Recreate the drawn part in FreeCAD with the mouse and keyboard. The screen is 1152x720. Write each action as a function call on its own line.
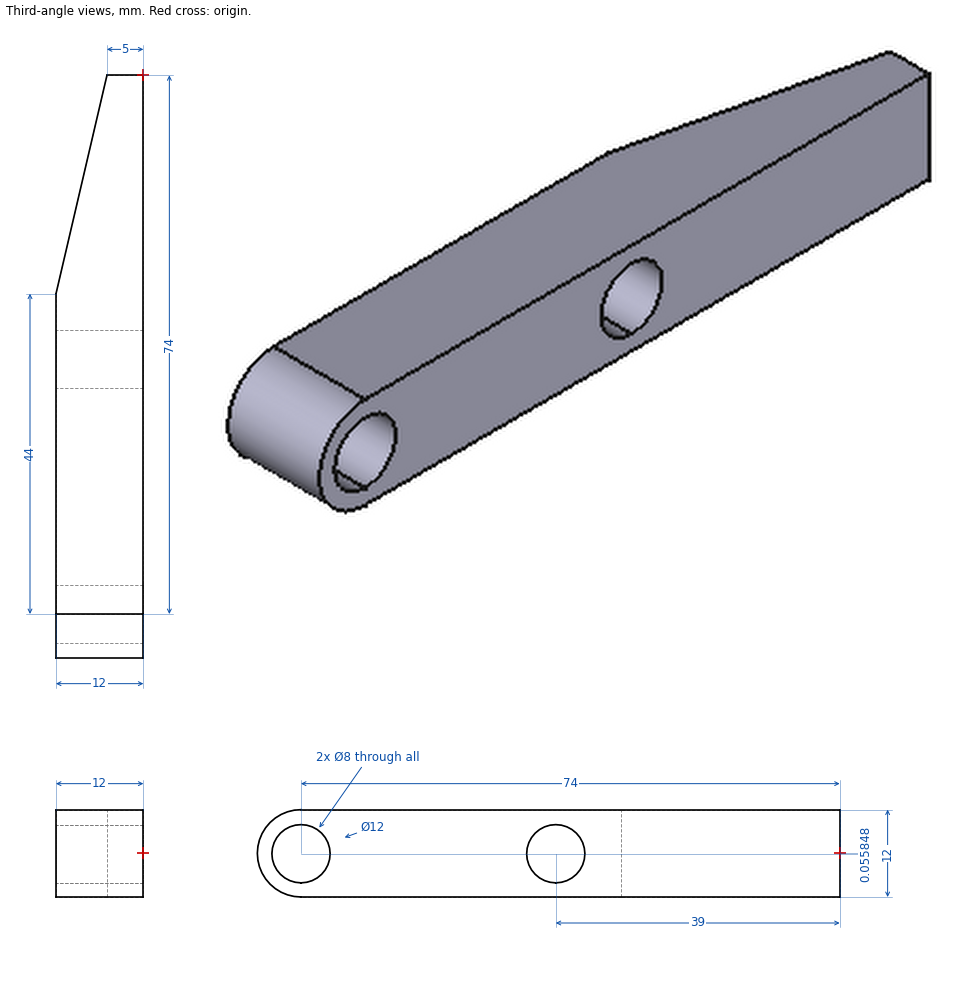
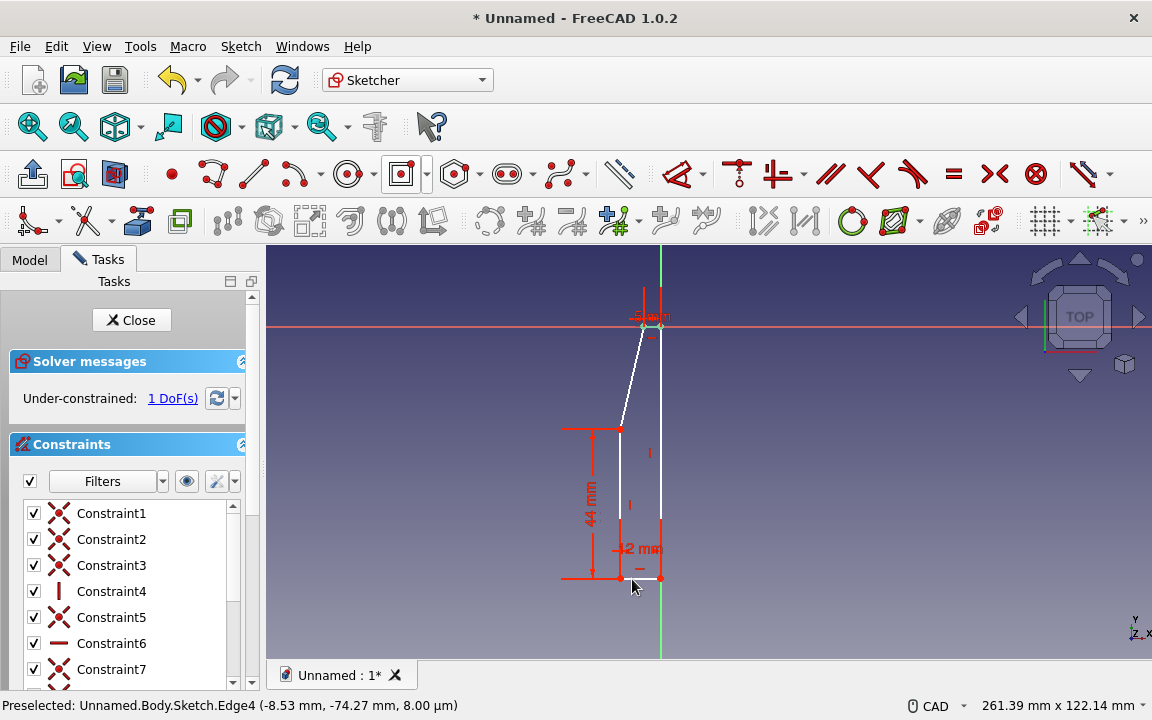
click(661, 503)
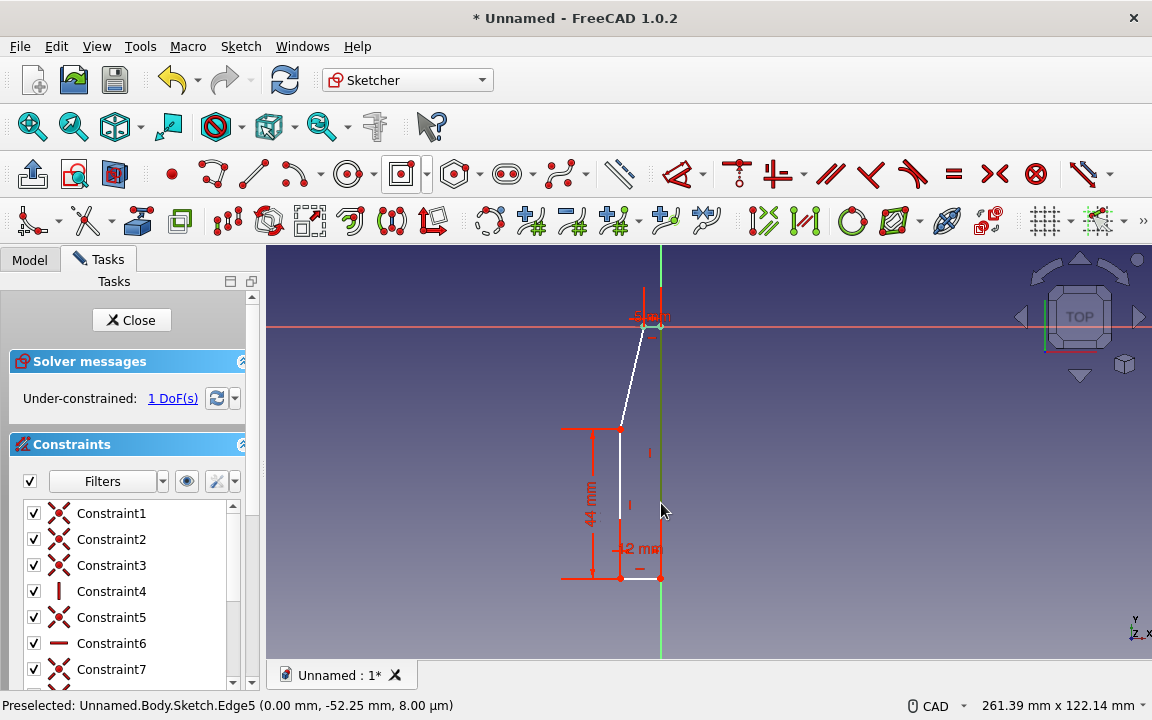
key(i)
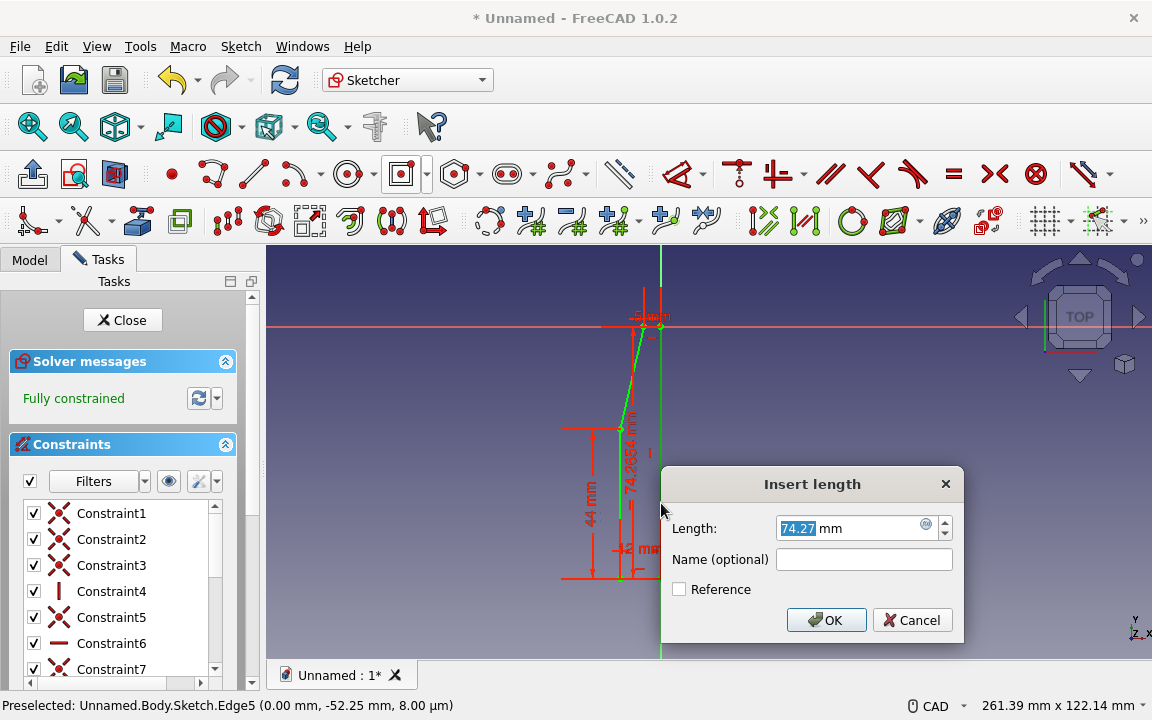
text(74)
key(Return)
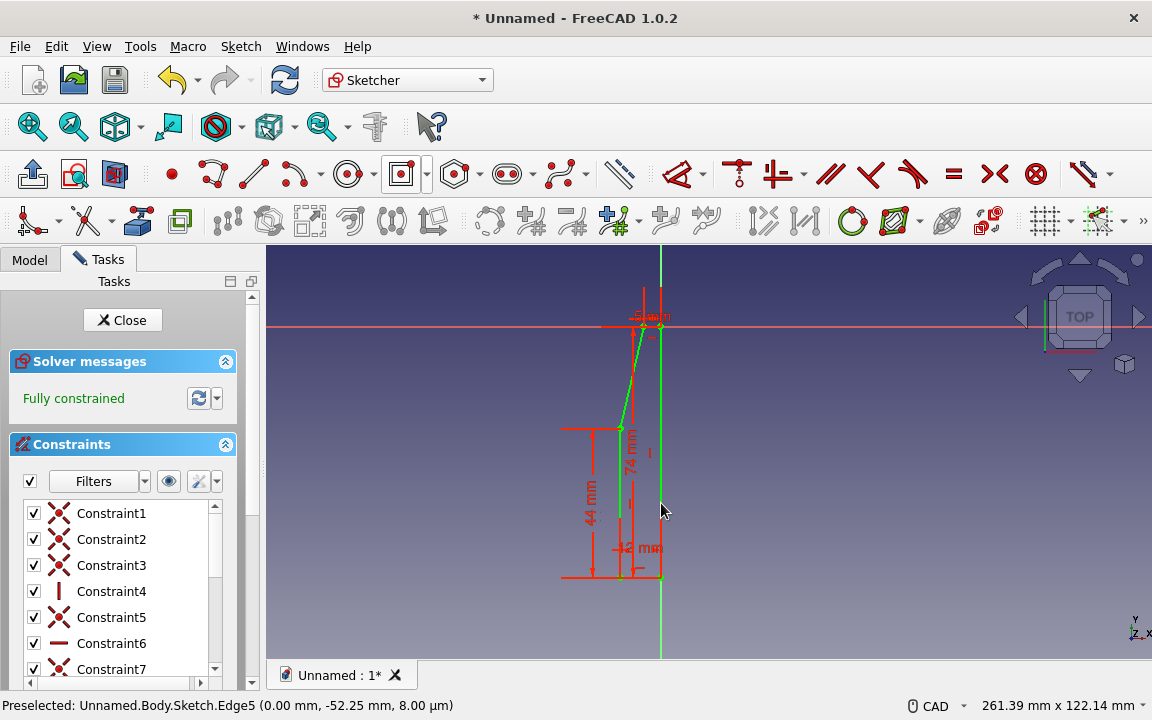
click(123, 320)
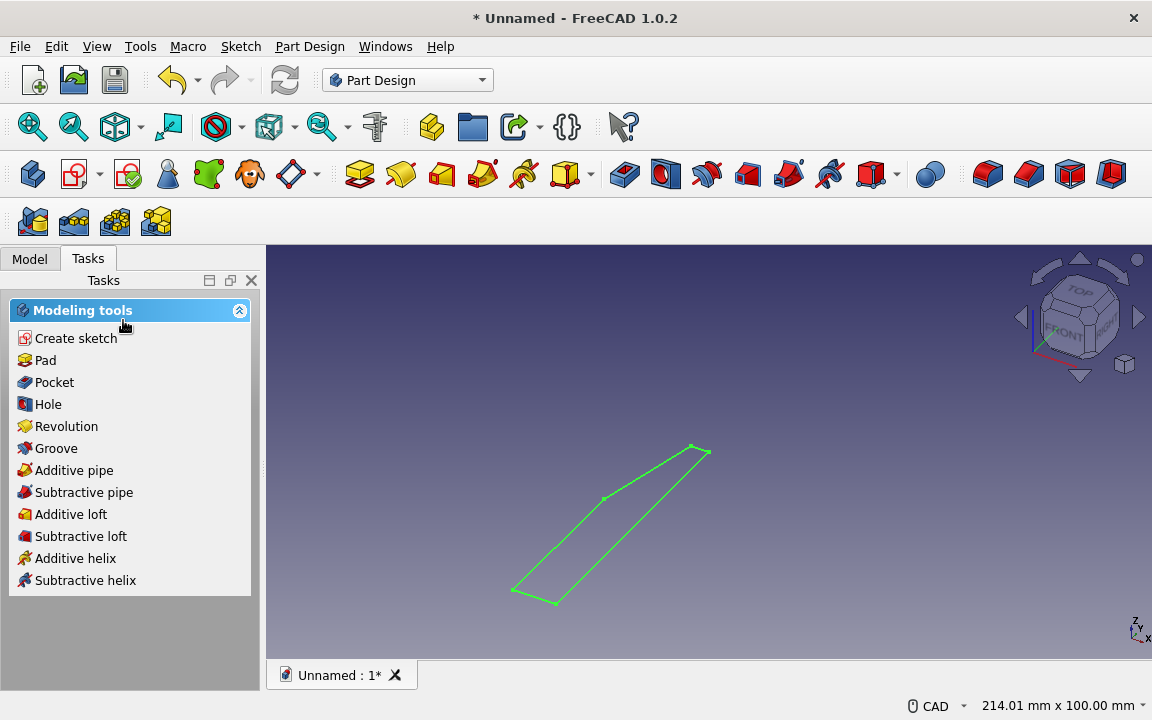
click(360, 174)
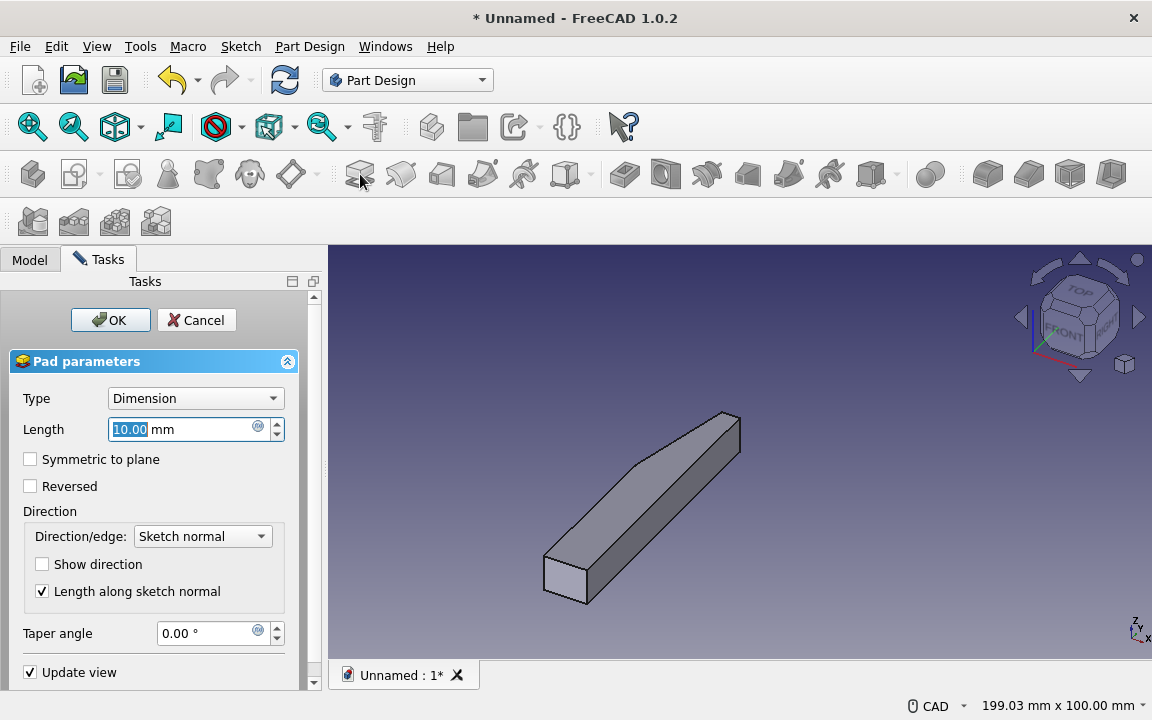
text(12)
key(Tab)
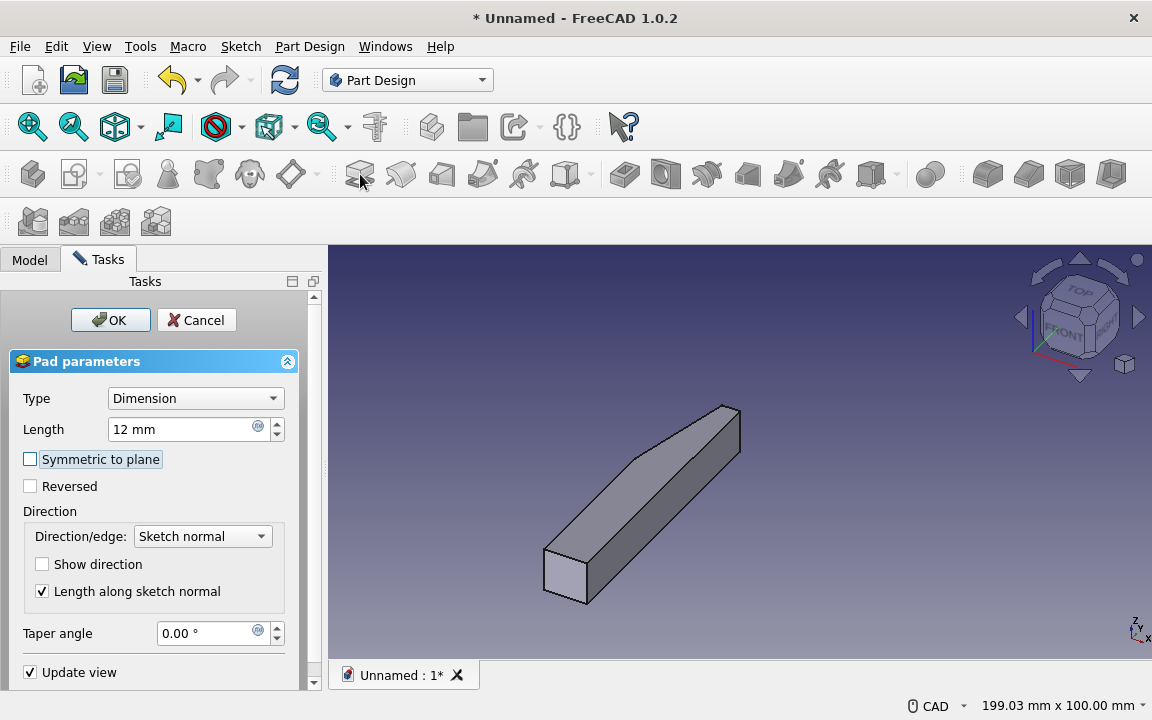
click(31, 459)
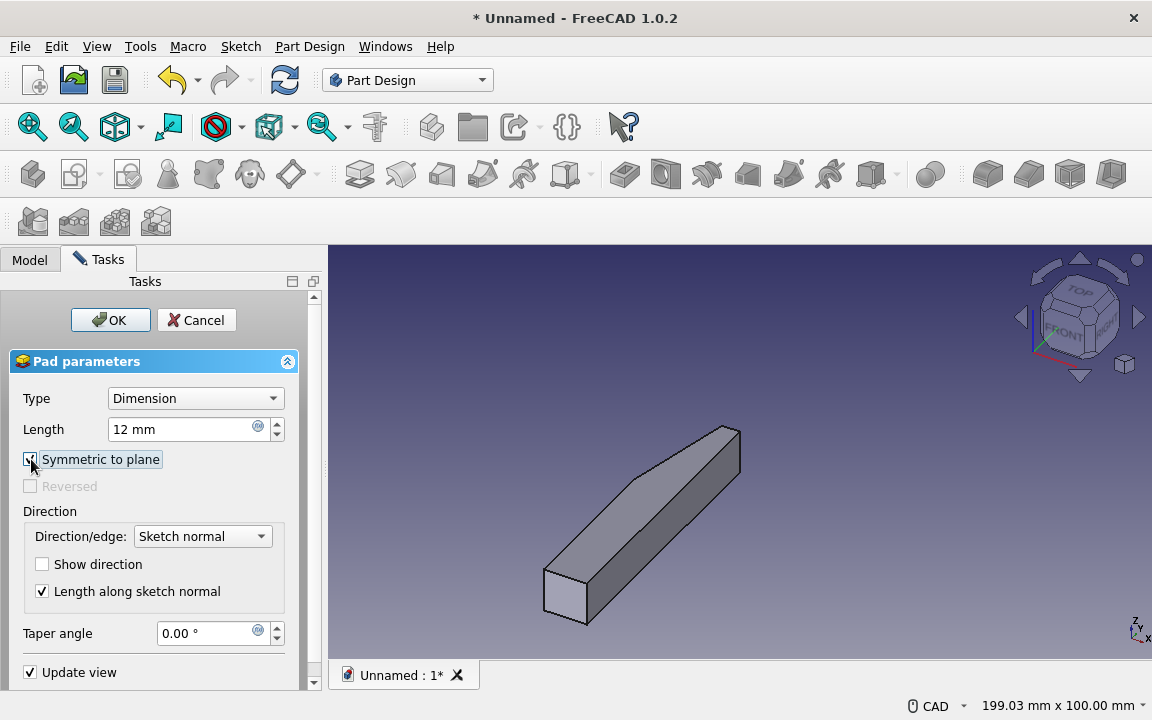
click(111, 320)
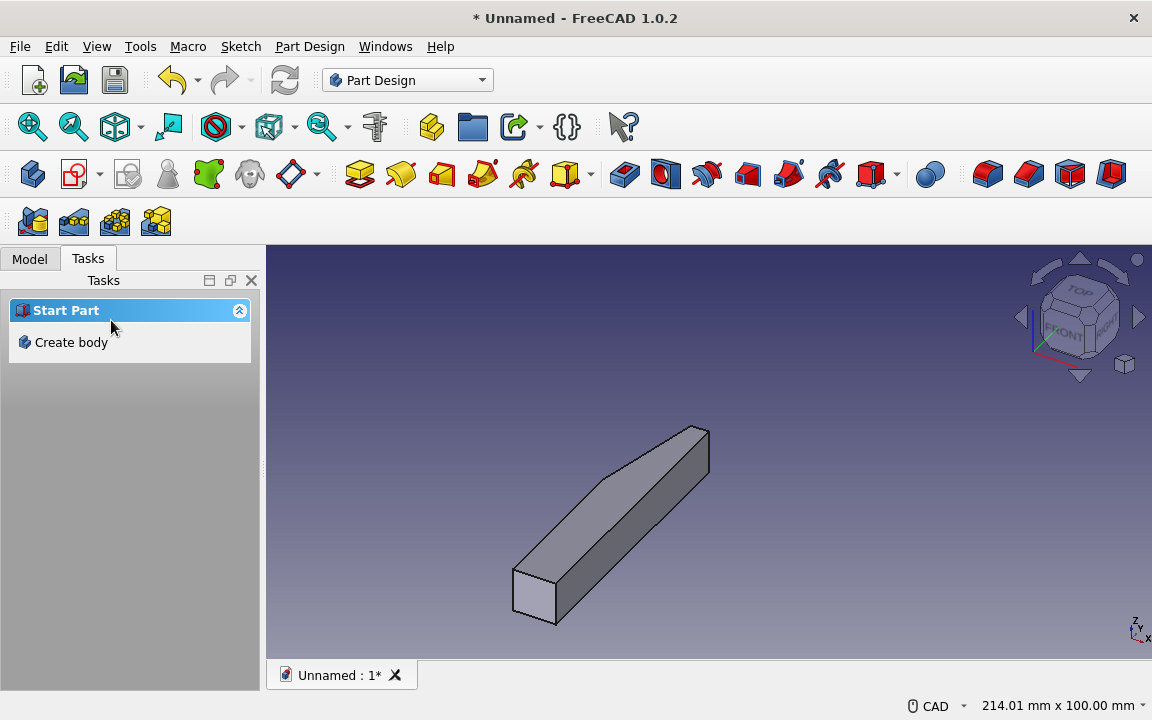
click(74, 174)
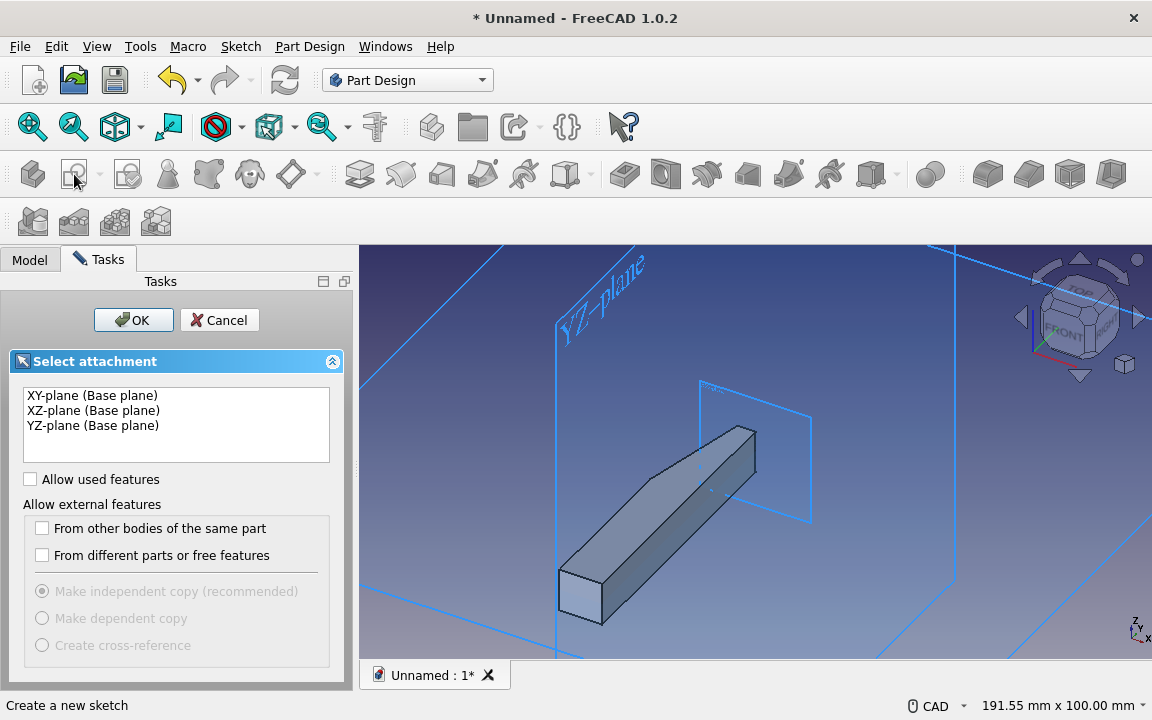
click(84, 426)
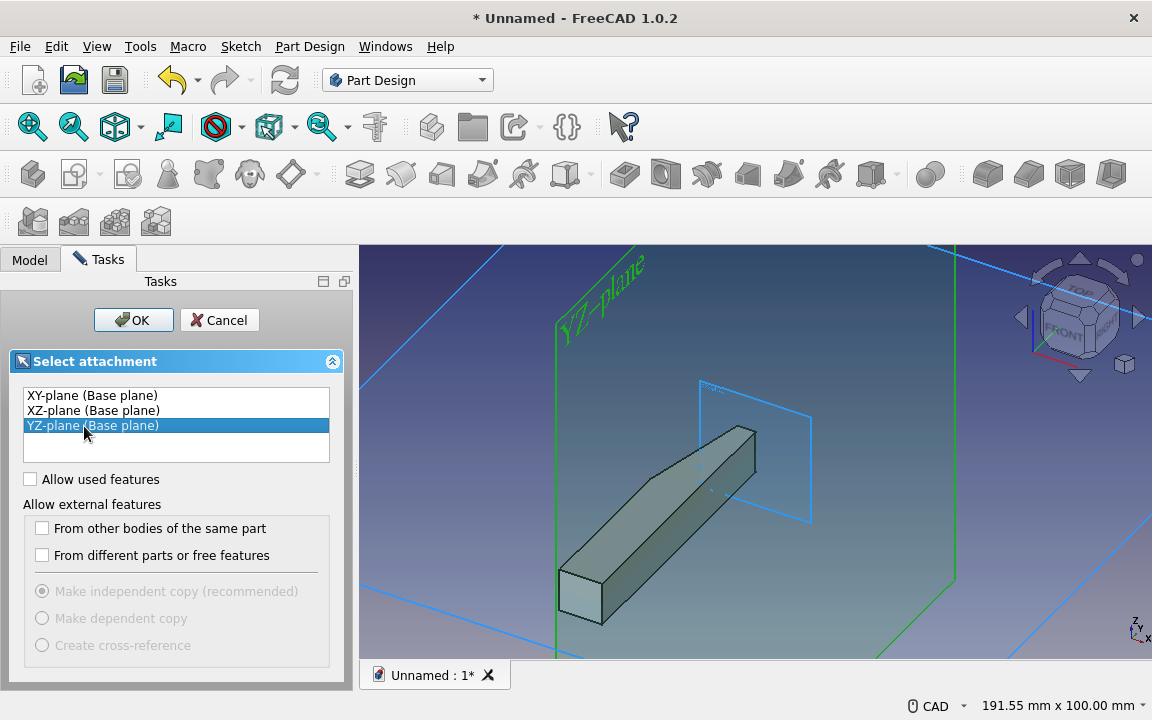
click(134, 320)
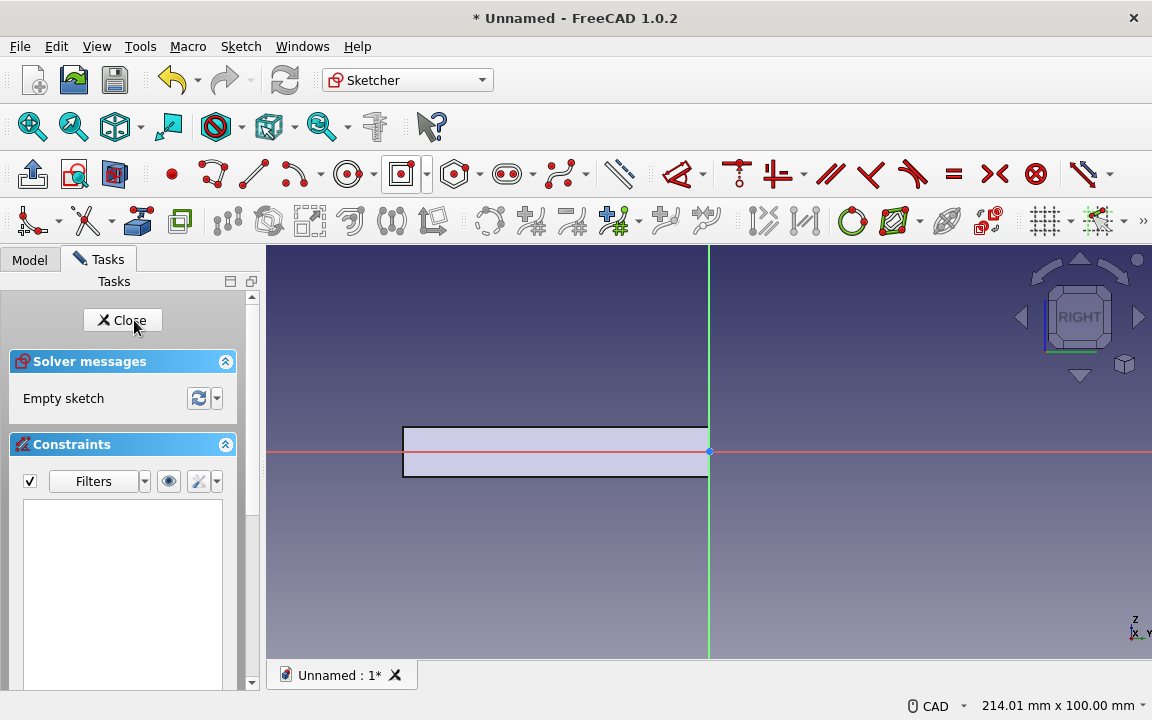
scroll(342, 452, up, 8)